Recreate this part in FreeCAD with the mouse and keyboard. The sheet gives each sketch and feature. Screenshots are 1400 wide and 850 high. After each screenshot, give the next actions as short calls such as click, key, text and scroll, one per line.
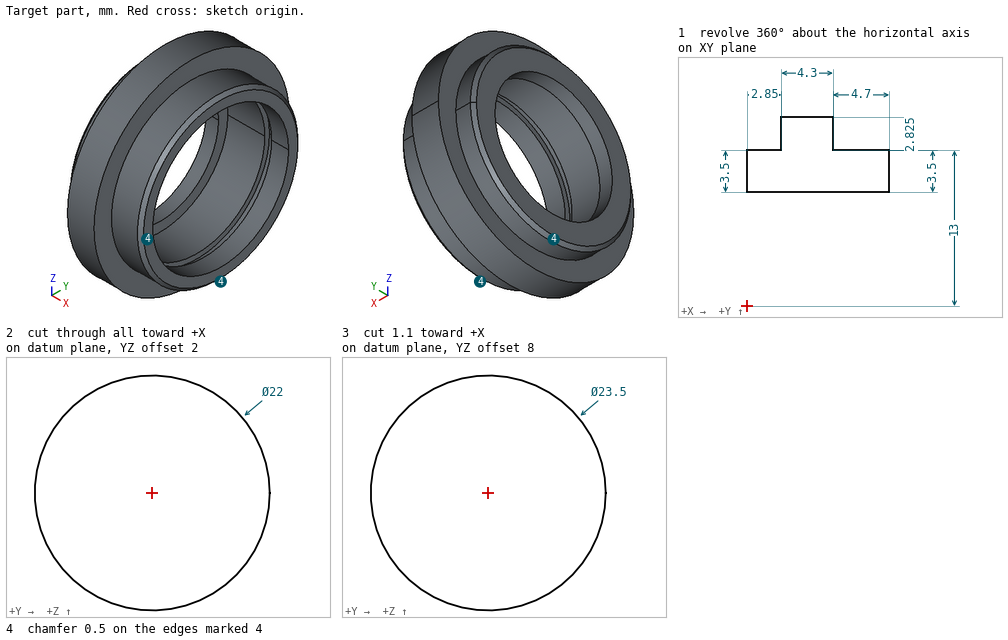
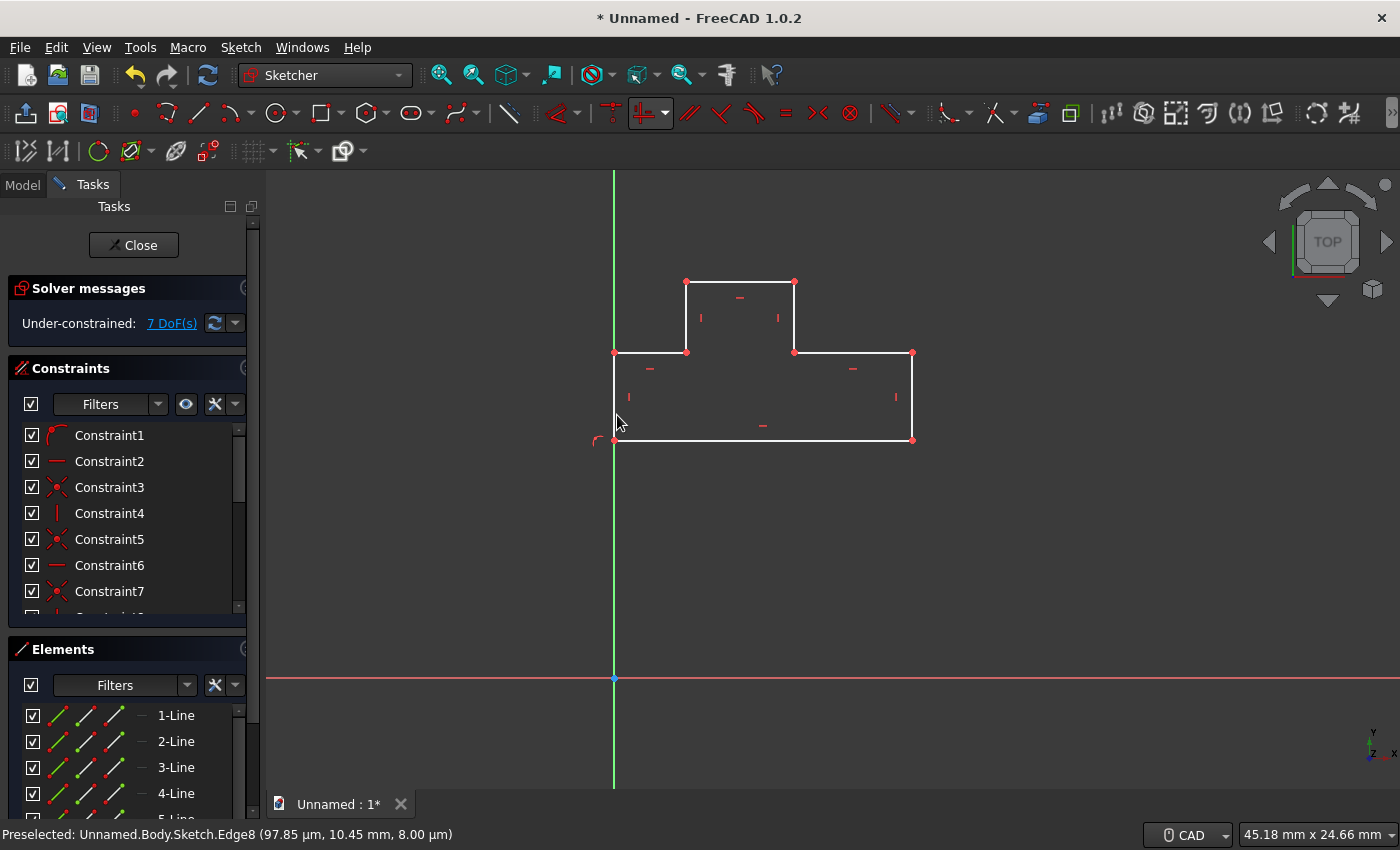
click(556, 114)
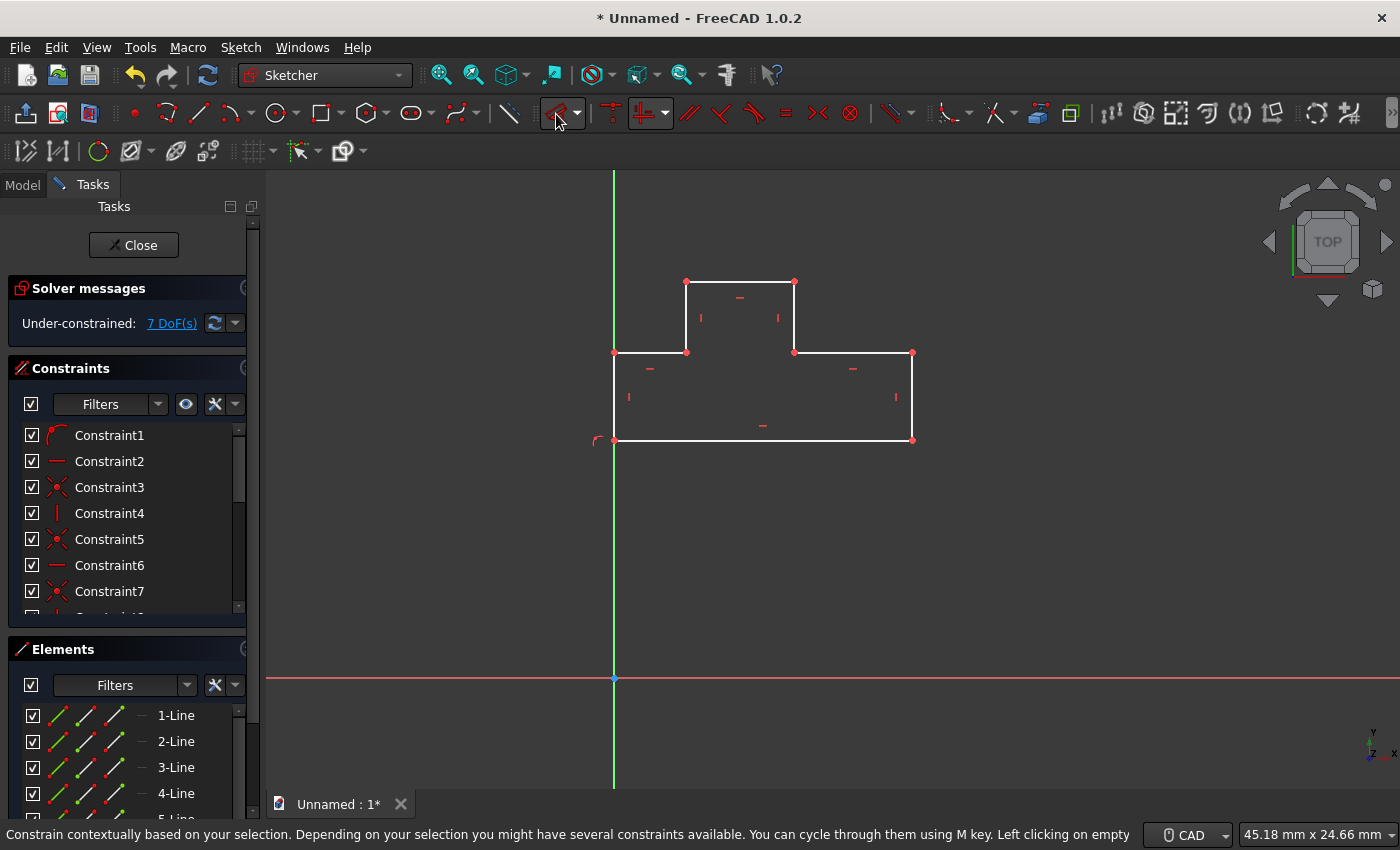
click(912, 415)
click(946, 397)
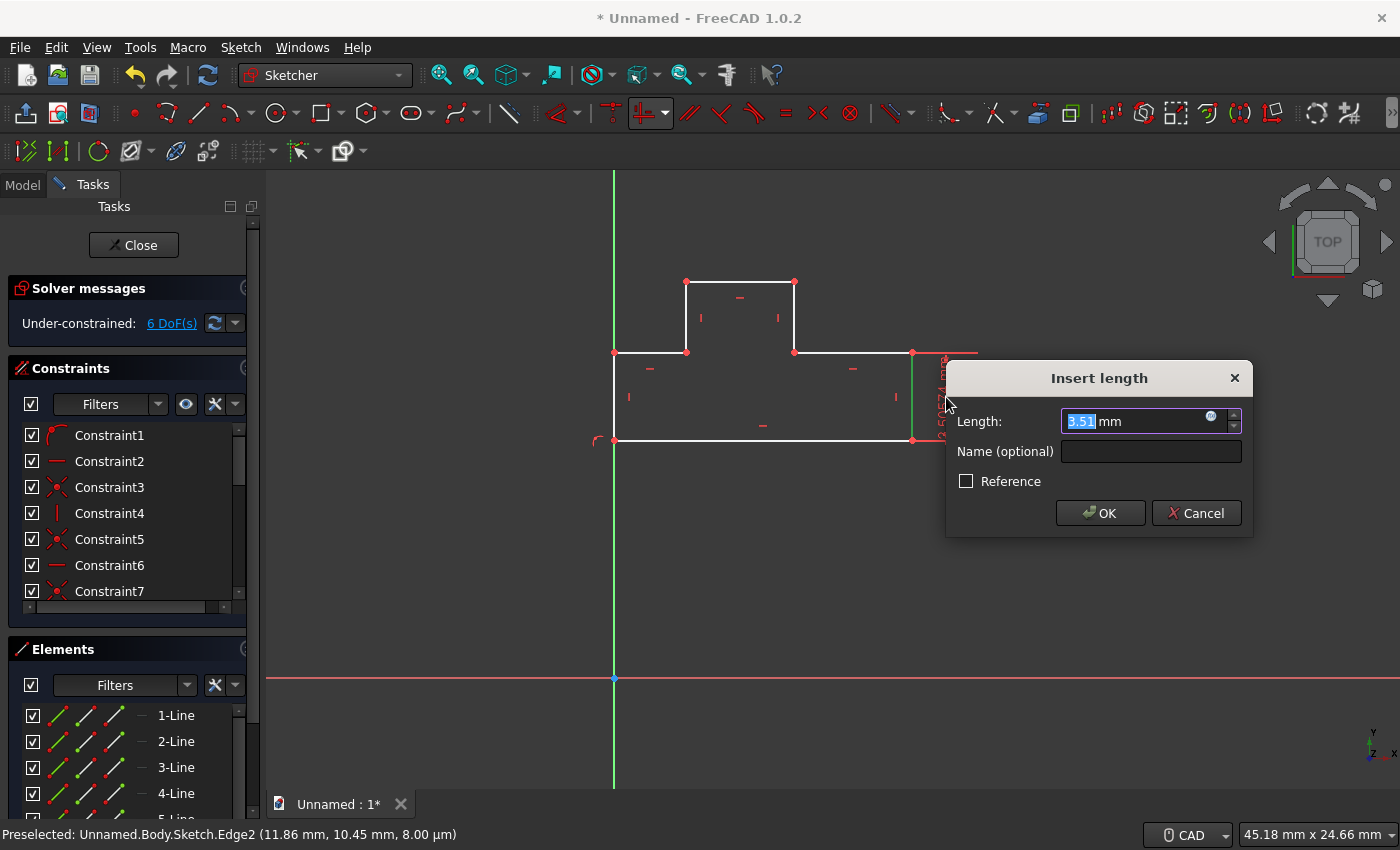
text(3.5)
key(Return)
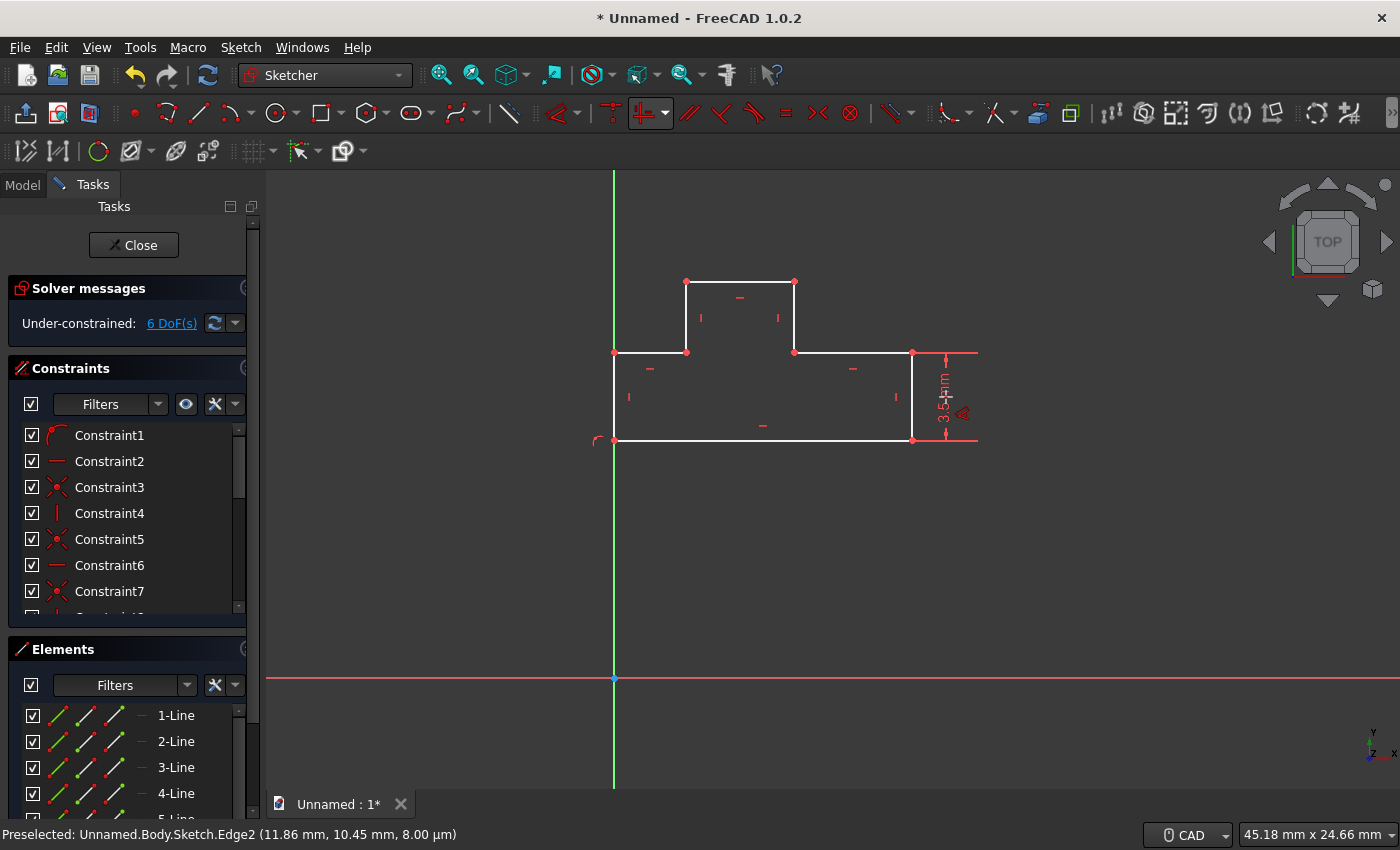
click(877, 353)
click(853, 319)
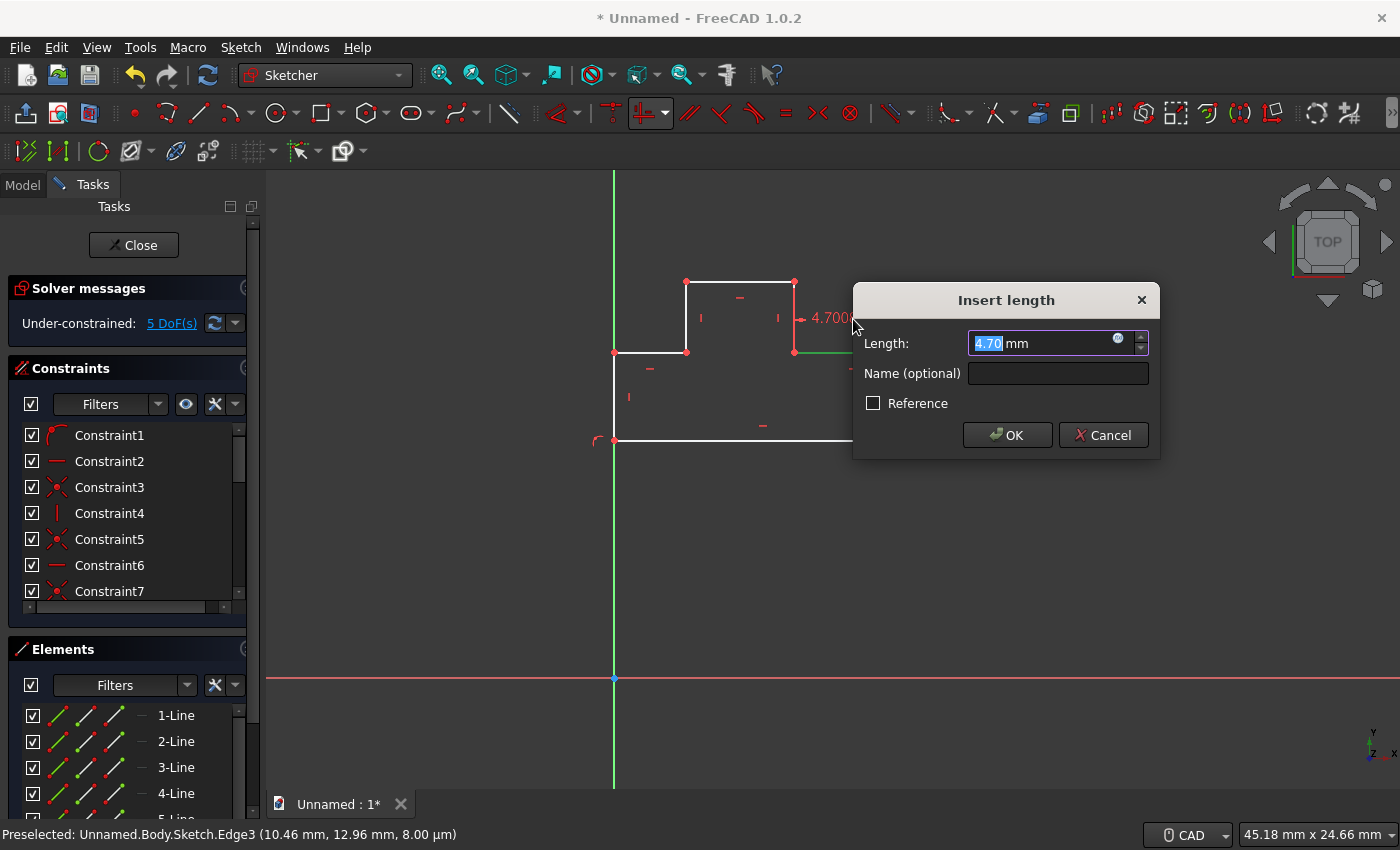
text(4.7)
key(Return)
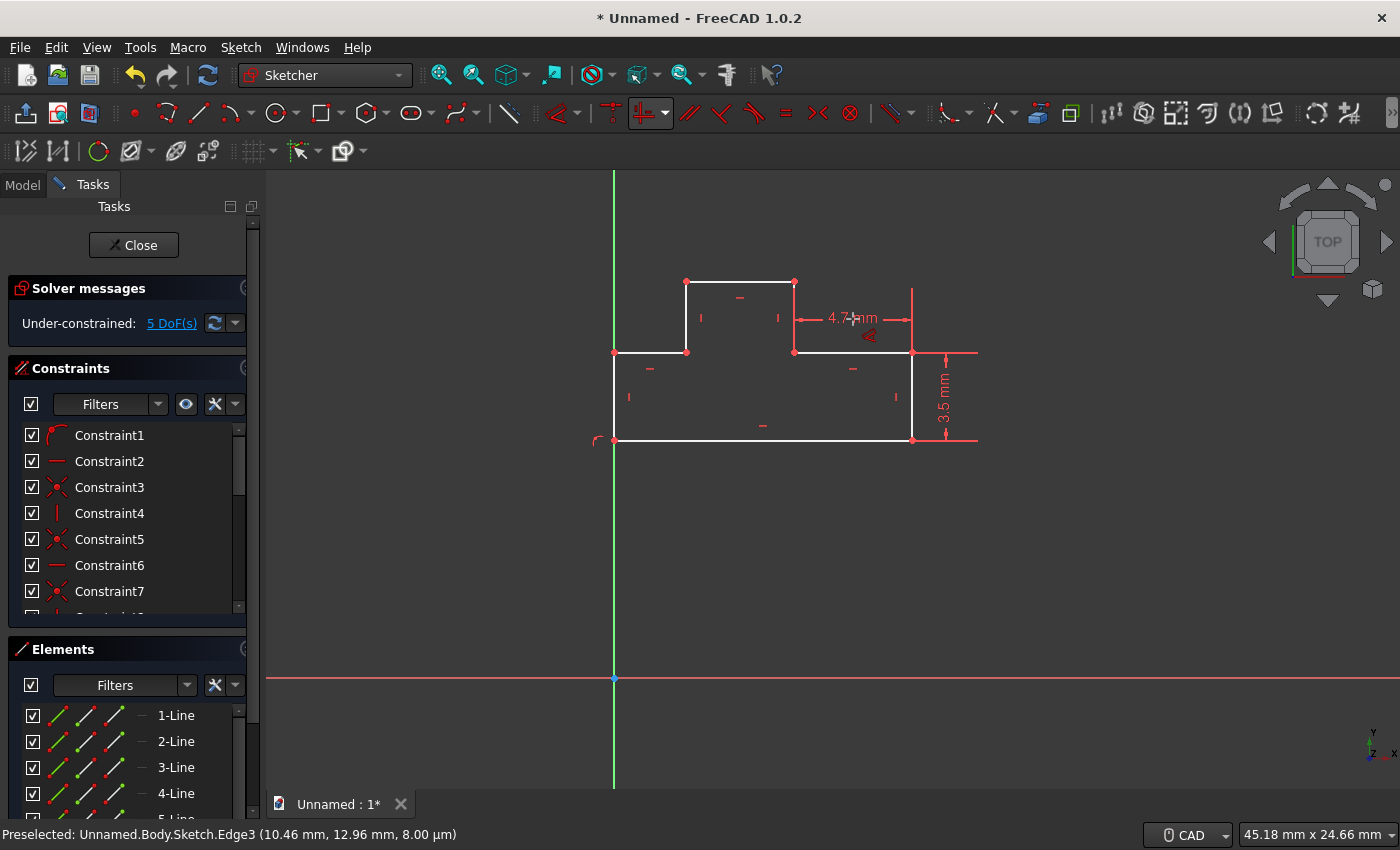
click(762, 282)
click(740, 248)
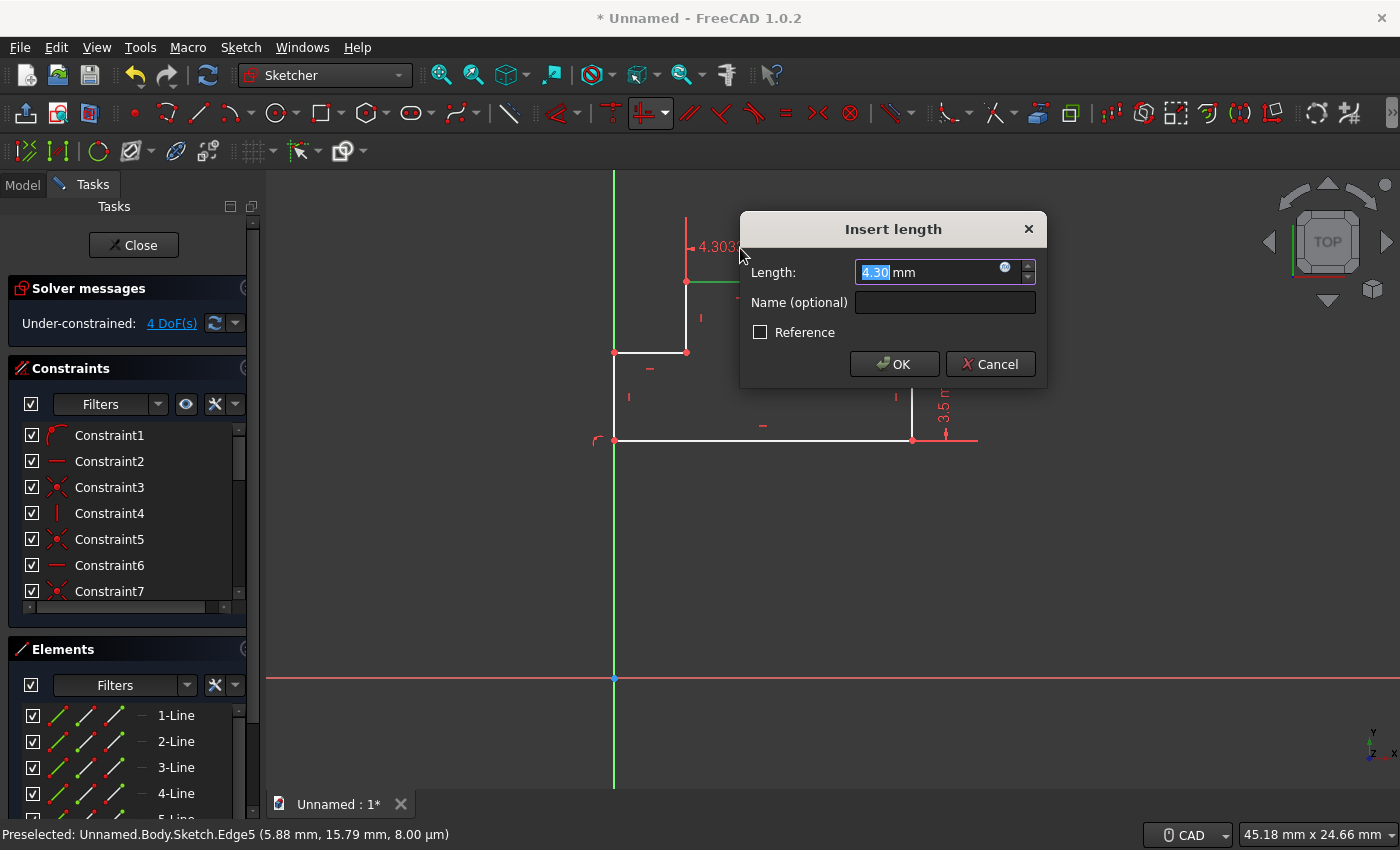
text(4.3)
key(Return)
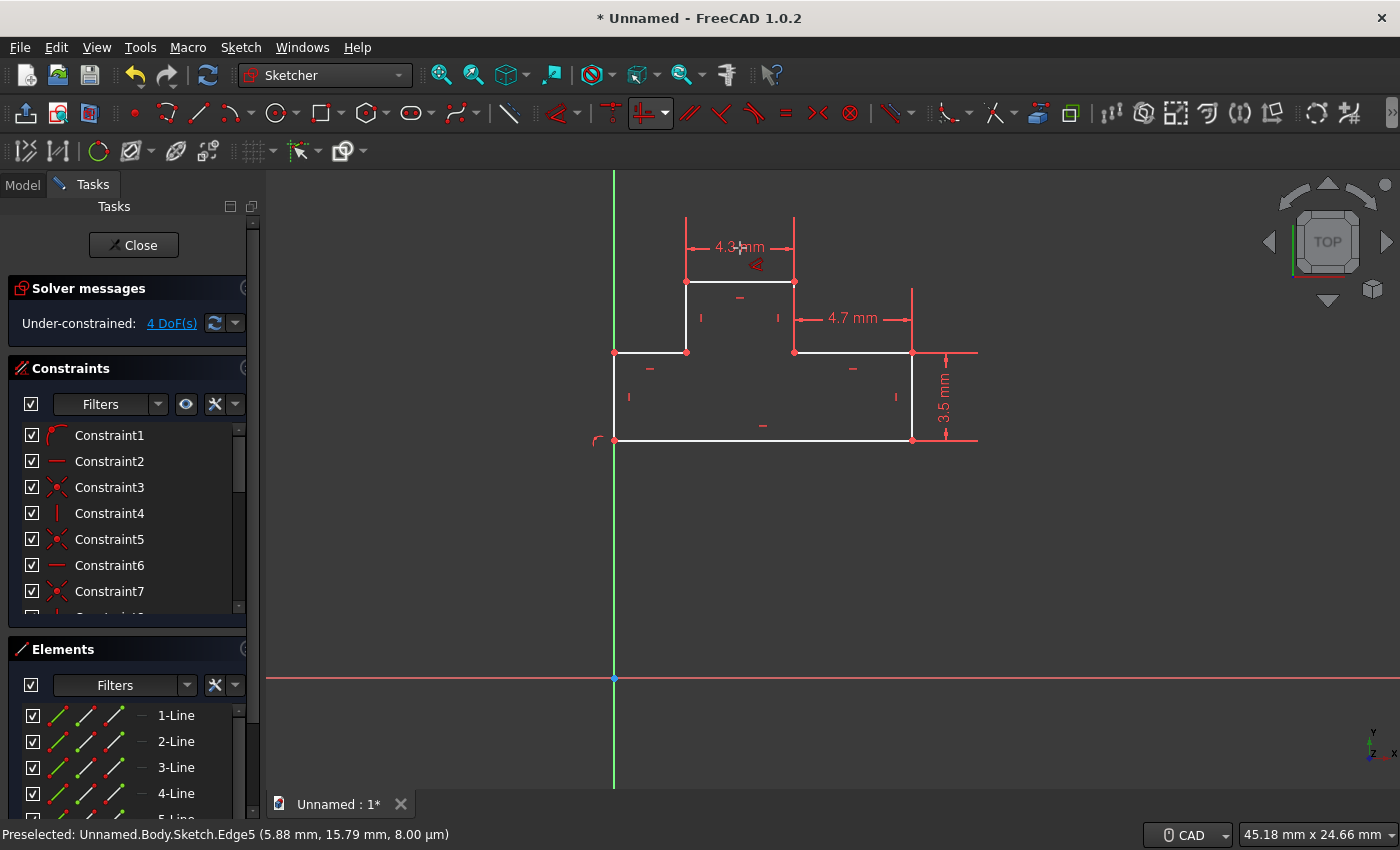
click(614, 379)
click(580, 397)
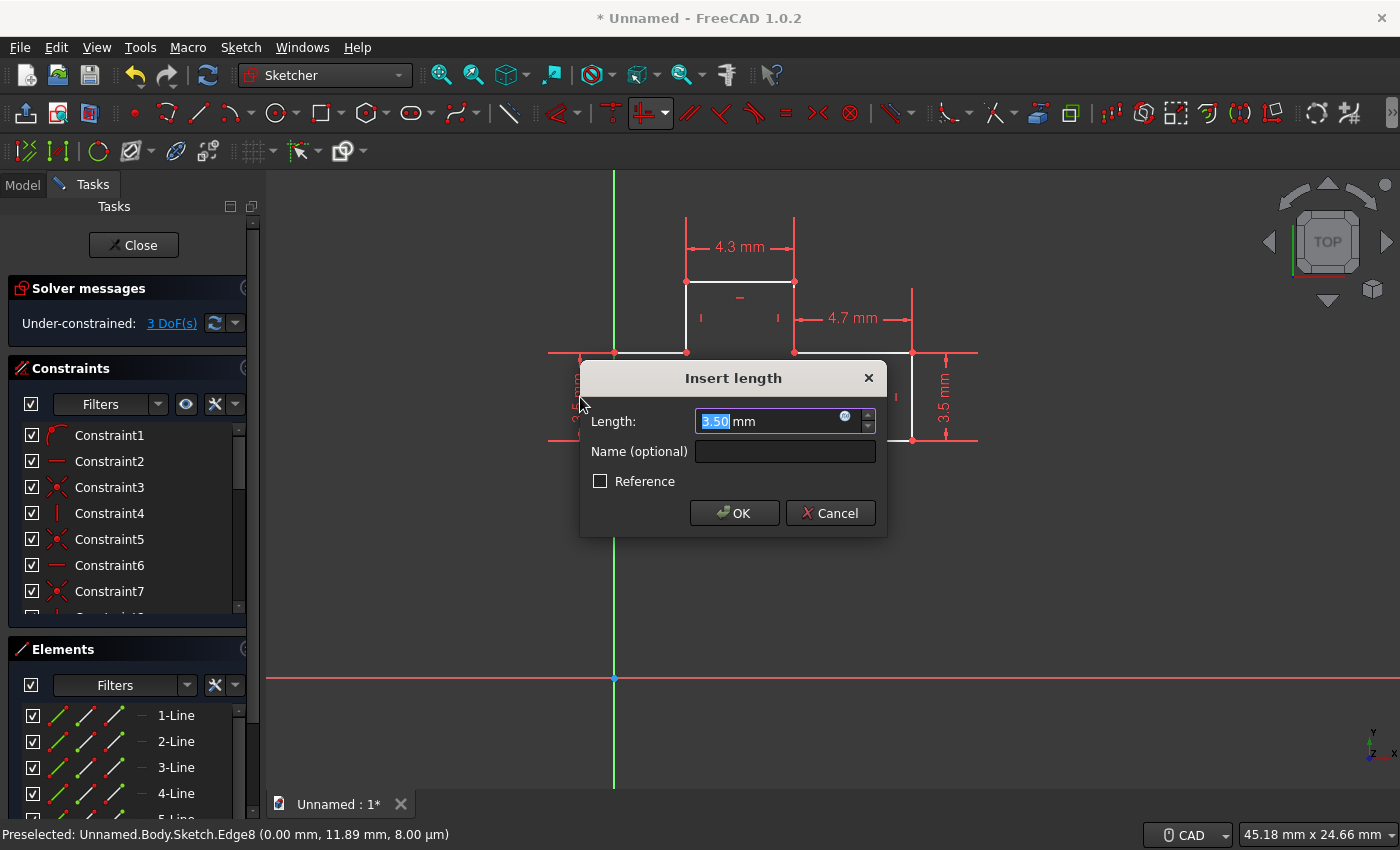
text(3.5)
key(Return)